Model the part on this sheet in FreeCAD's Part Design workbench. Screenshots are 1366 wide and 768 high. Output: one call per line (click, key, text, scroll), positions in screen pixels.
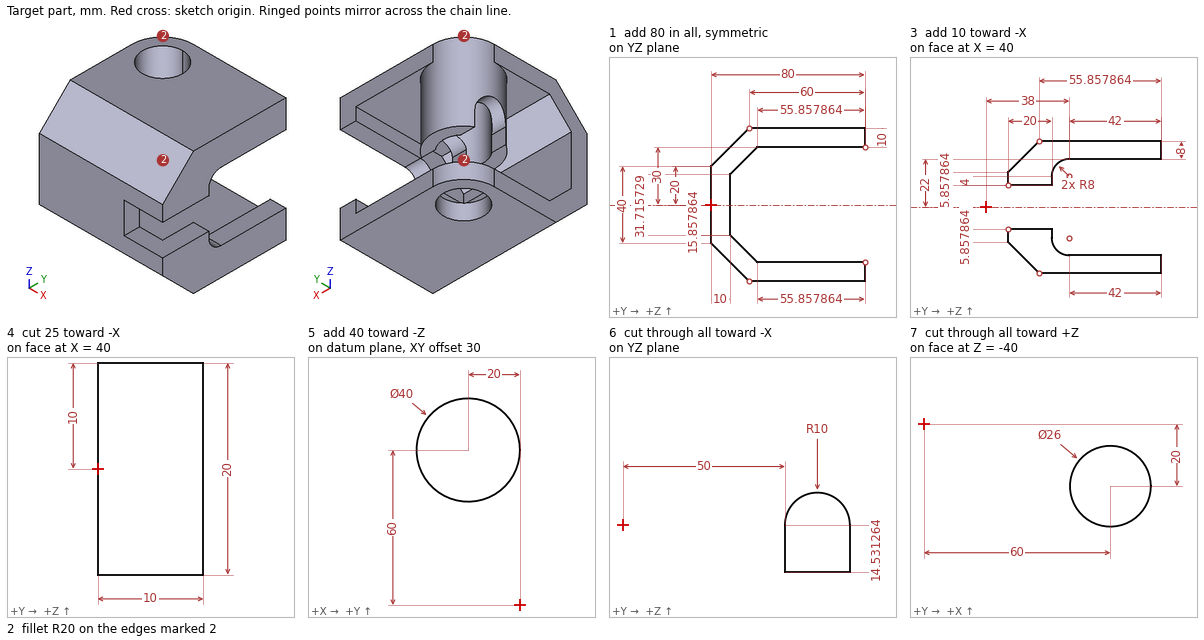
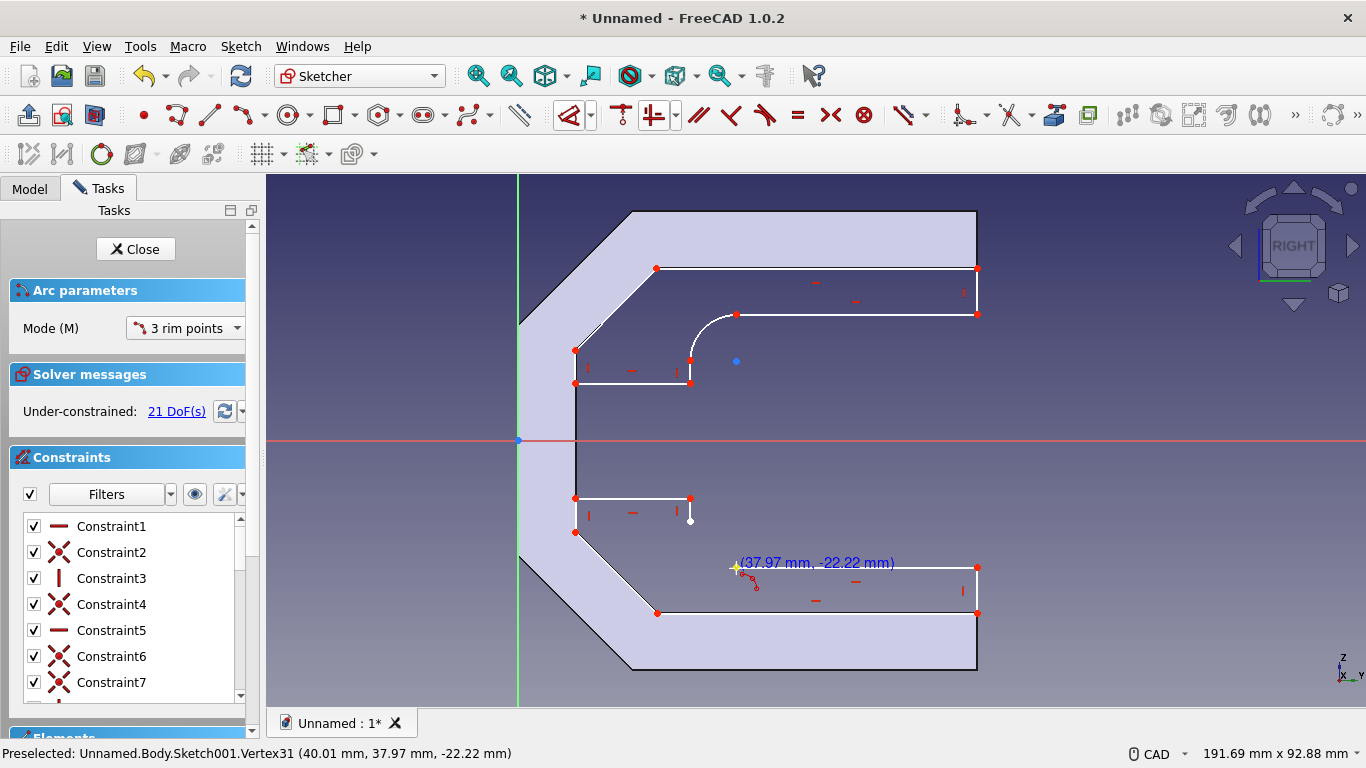
scroll(690, 521, up, 2)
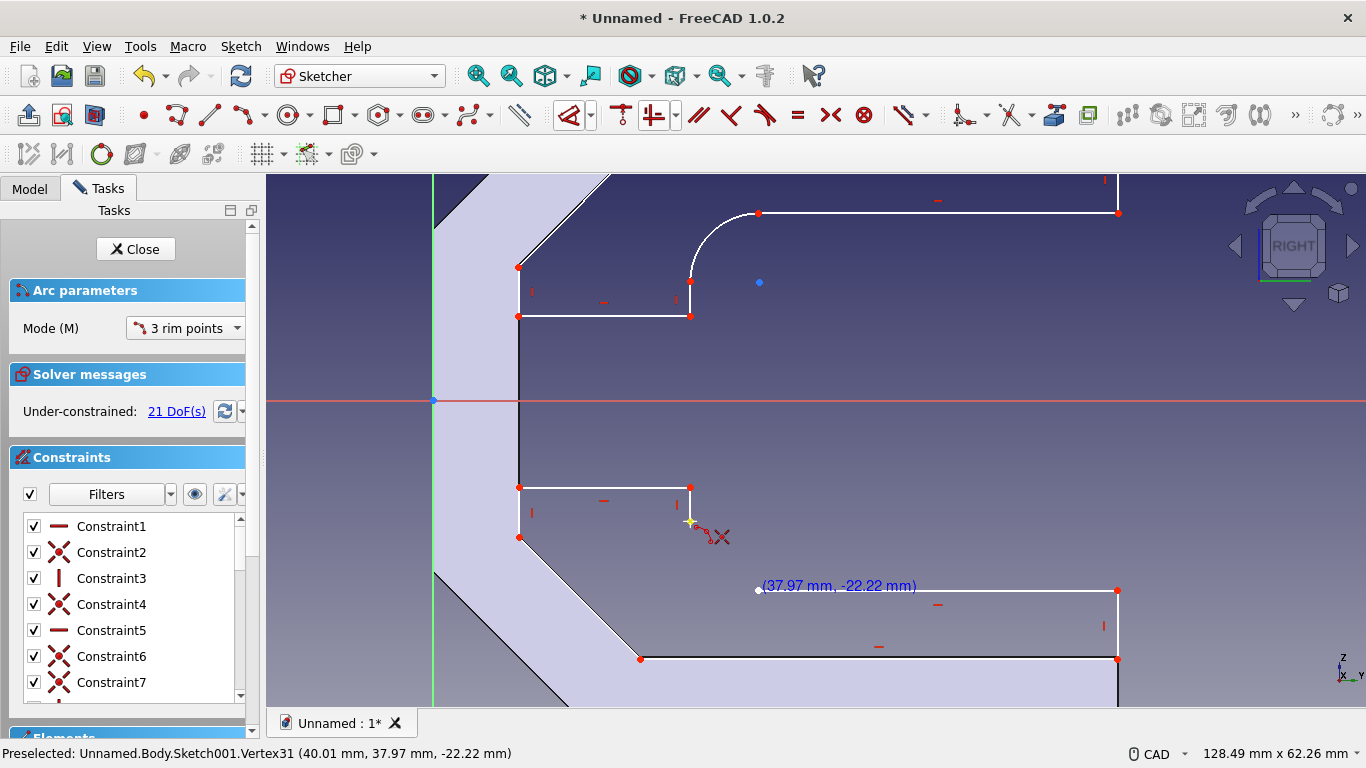
click(690, 522)
click(710, 569)
key(Escape)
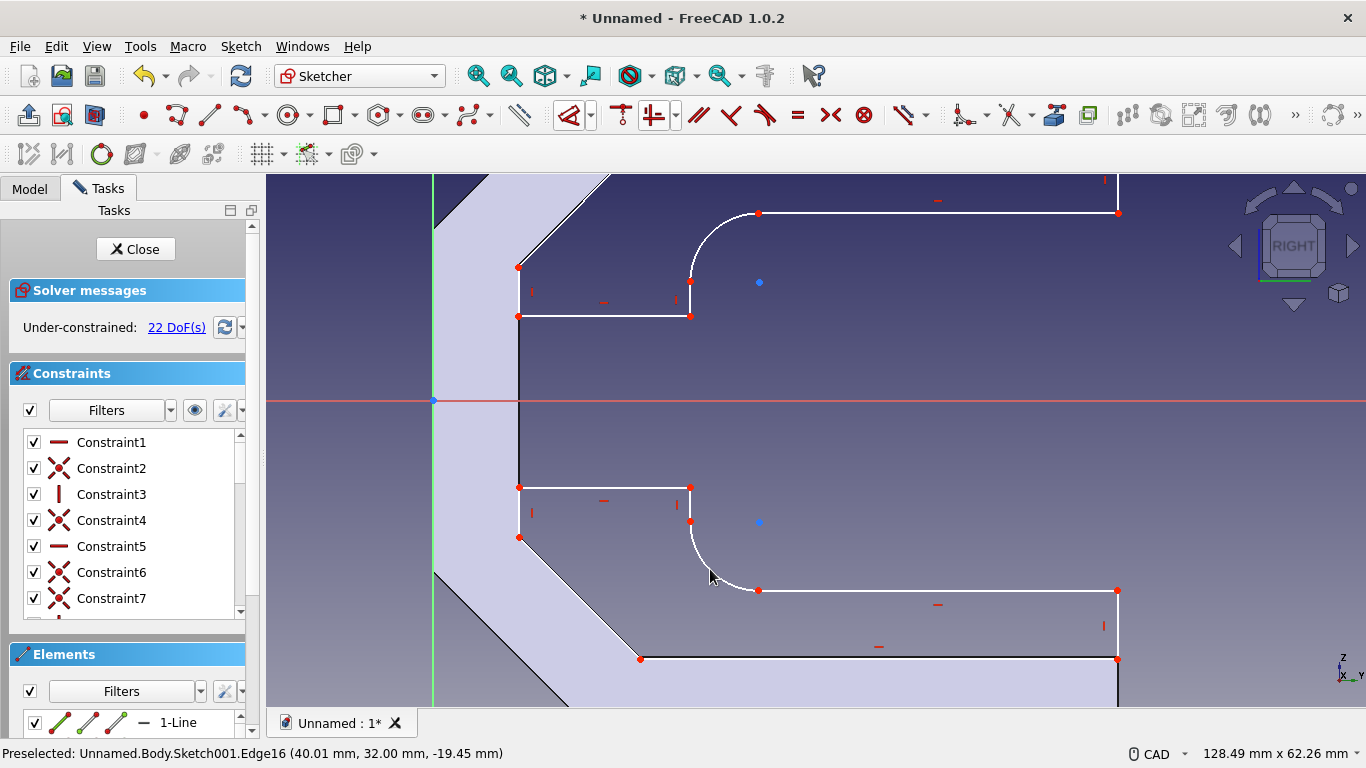
click(867, 213)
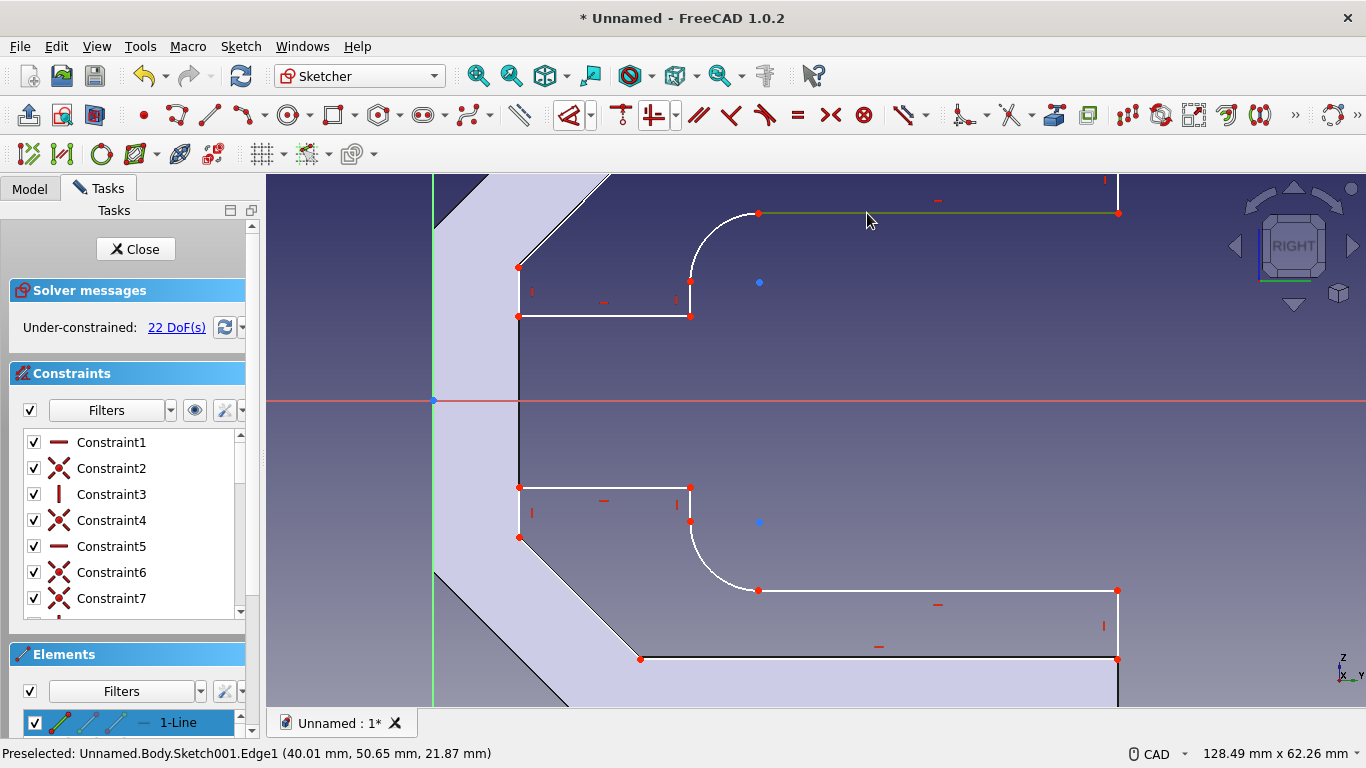
click(728, 221)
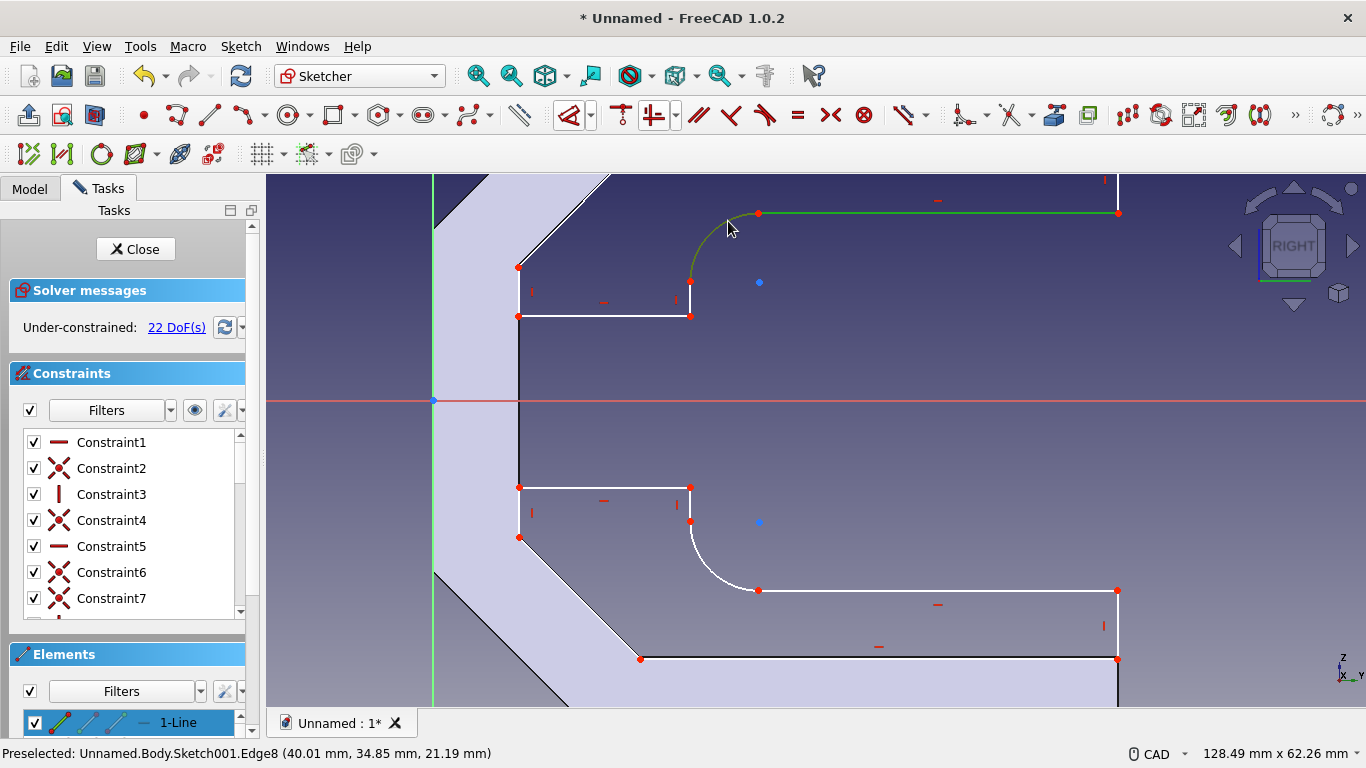
click(765, 116)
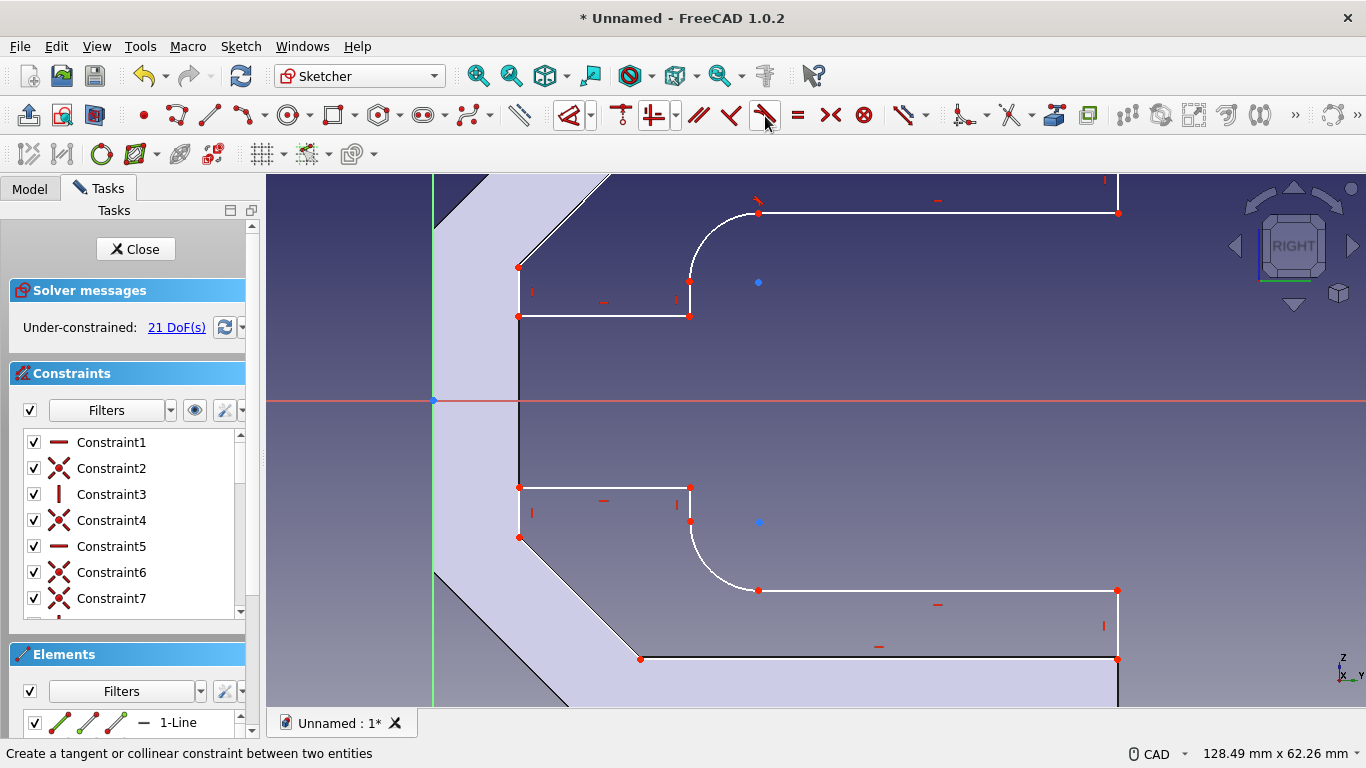
scroll(690, 306, up, 2)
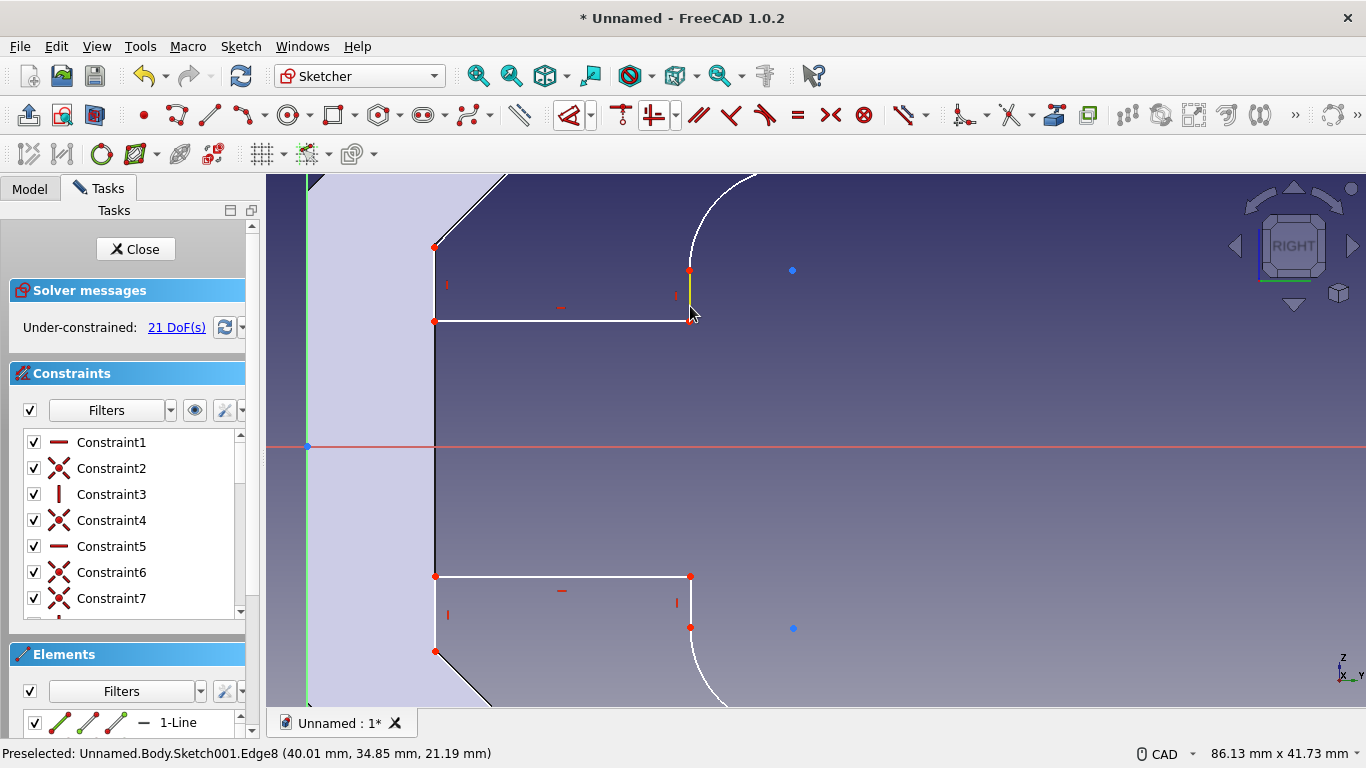
click(690, 306)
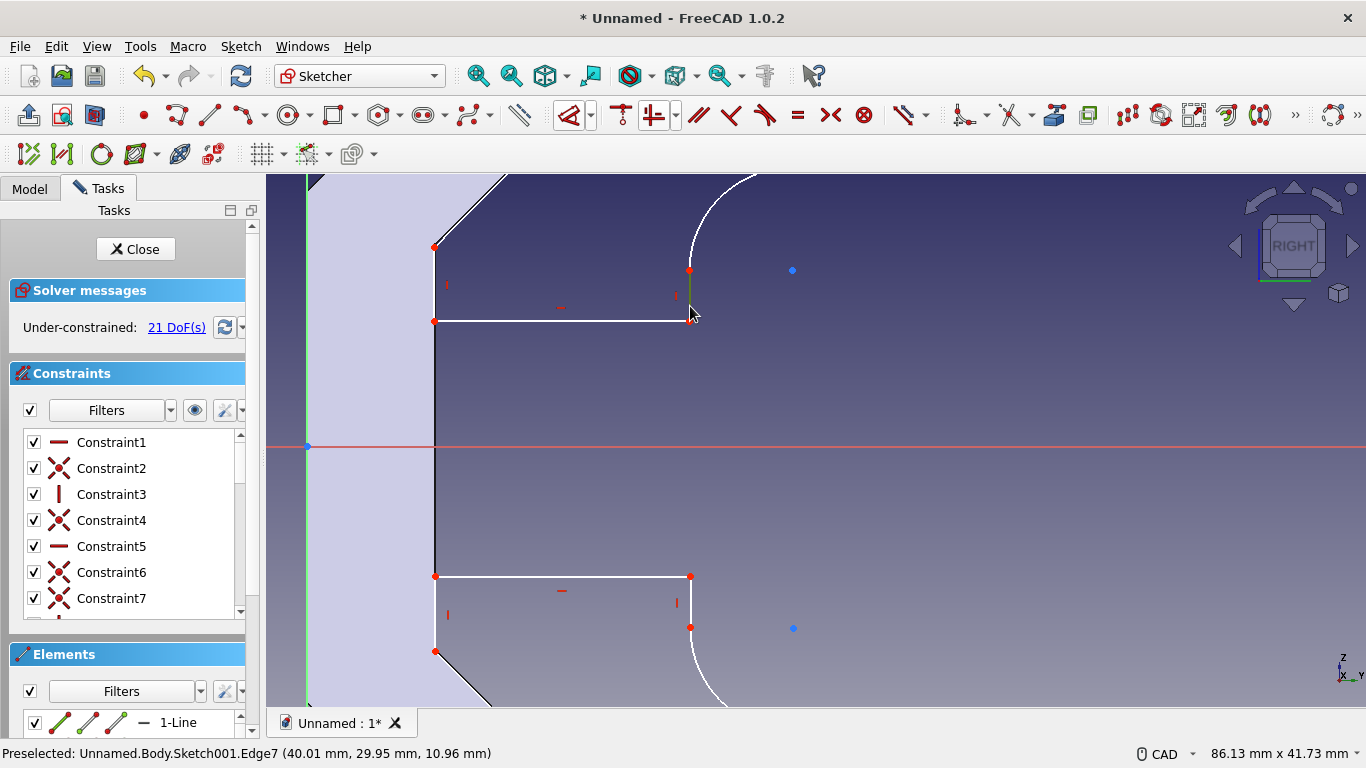
click(701, 224)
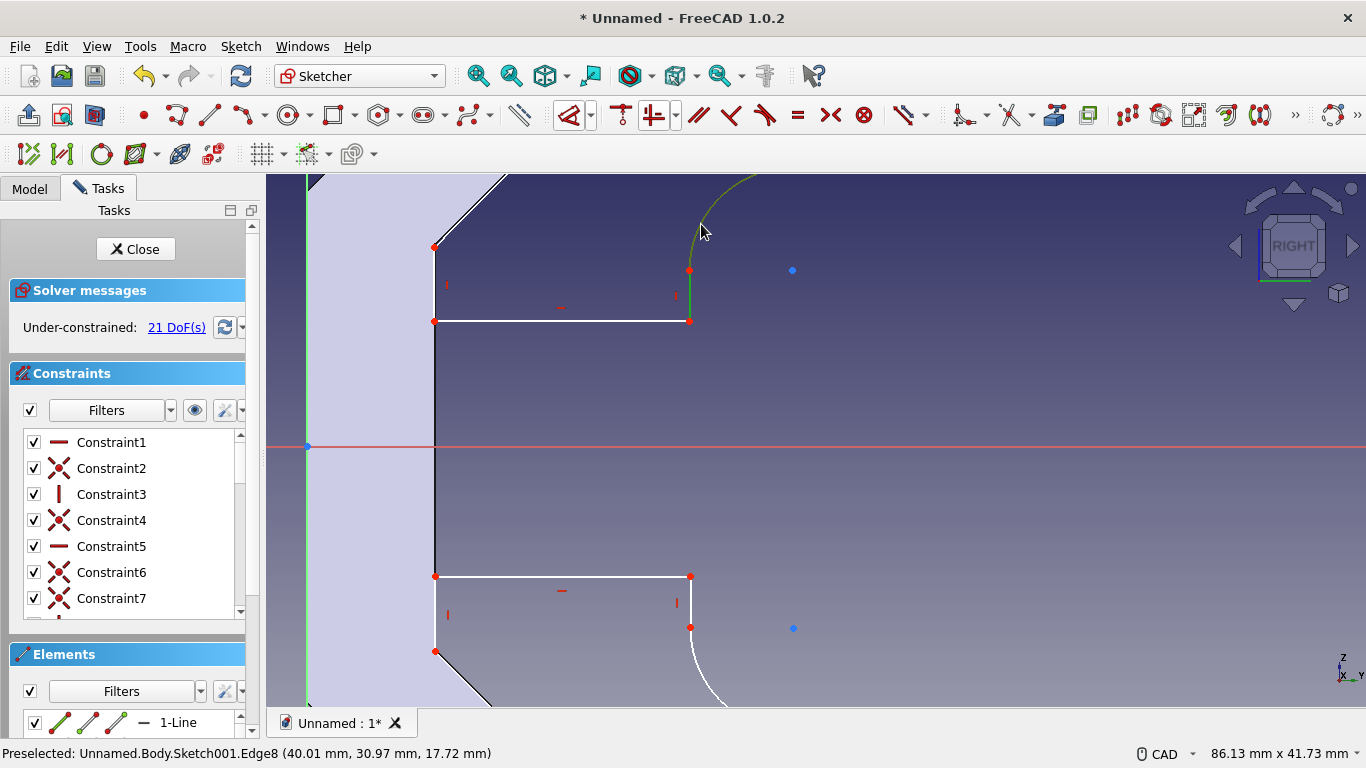
key(t)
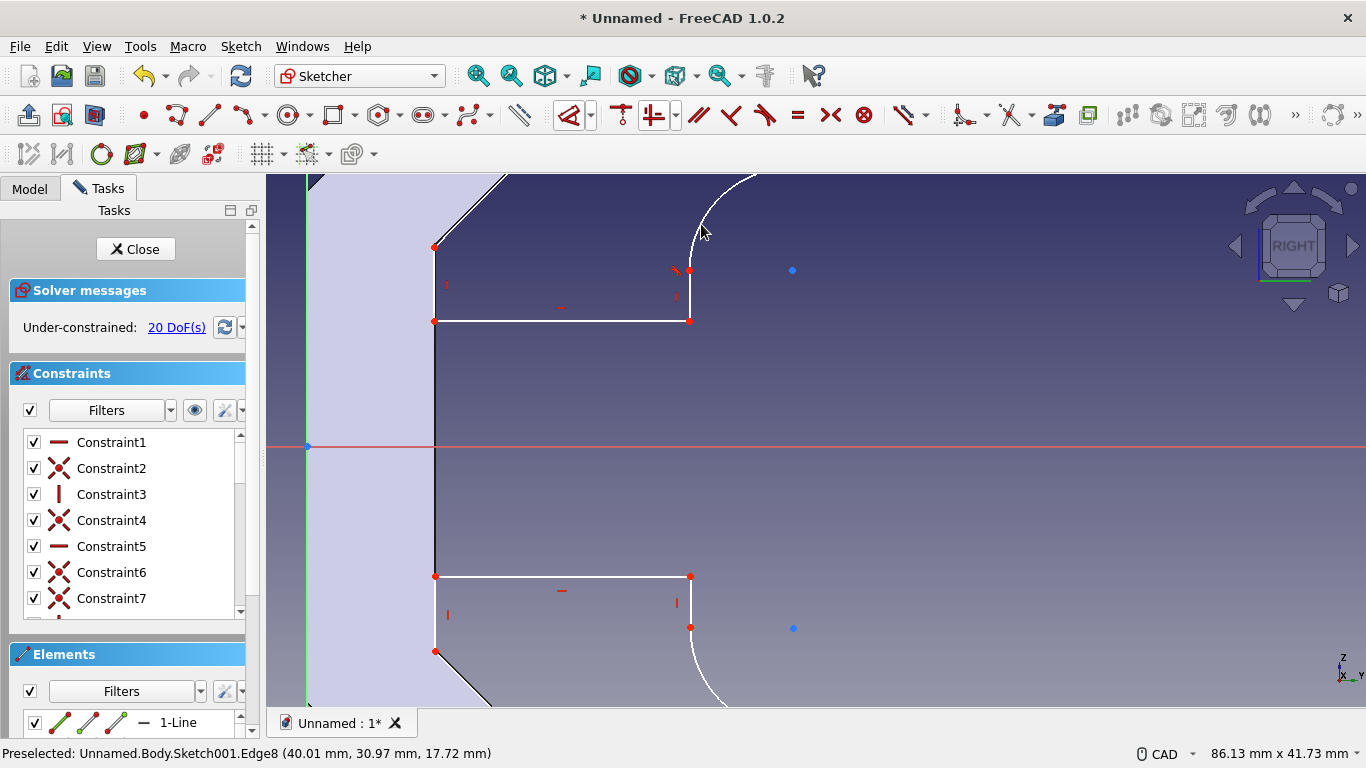
click(691, 612)